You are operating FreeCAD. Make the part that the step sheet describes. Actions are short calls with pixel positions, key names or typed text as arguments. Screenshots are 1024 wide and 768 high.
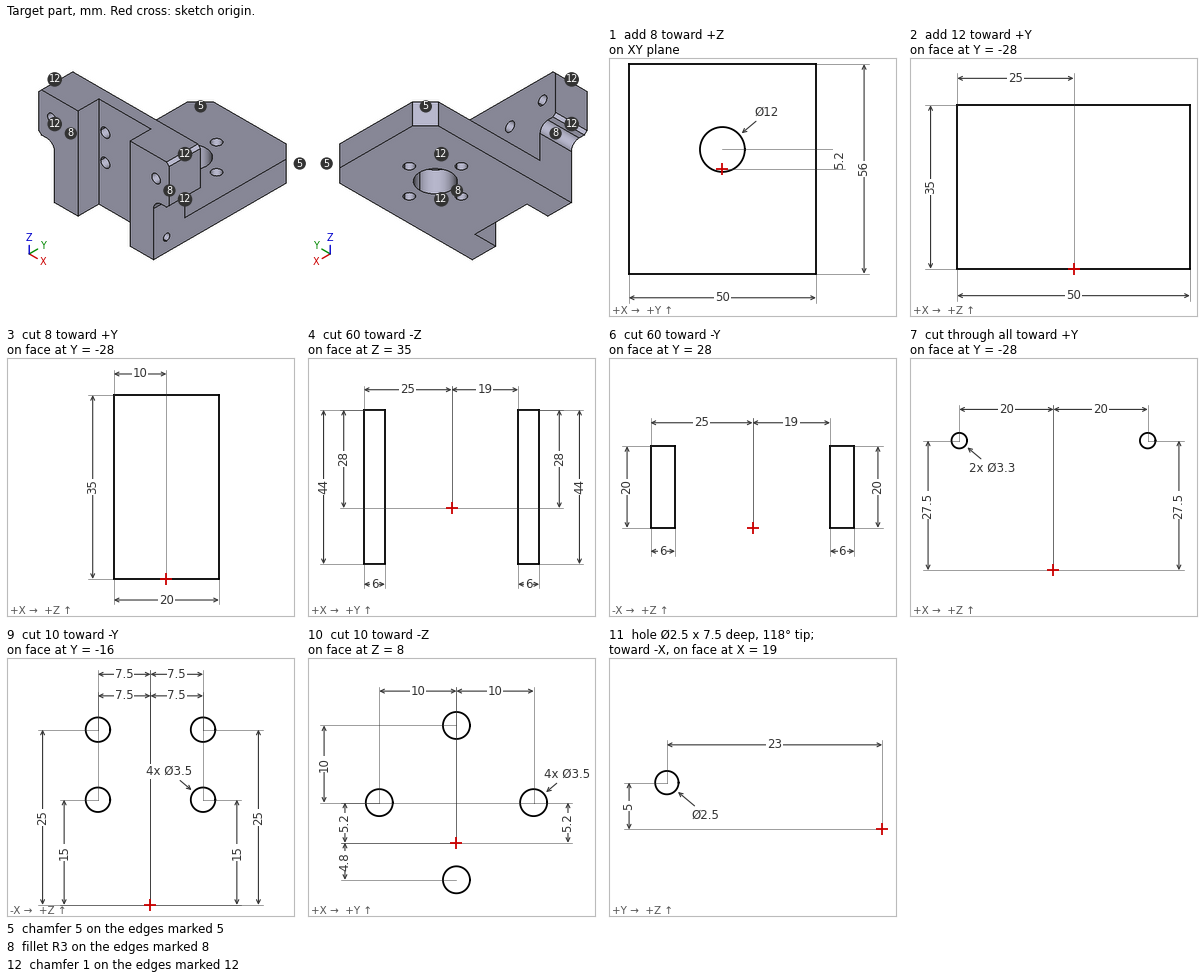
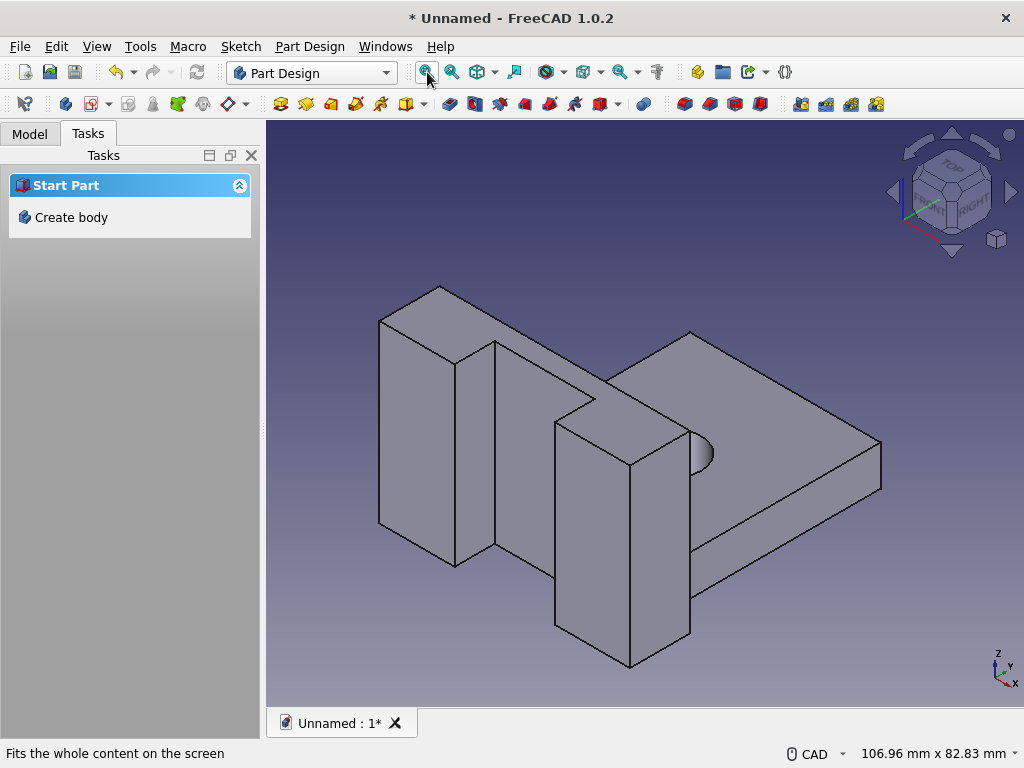
key(2)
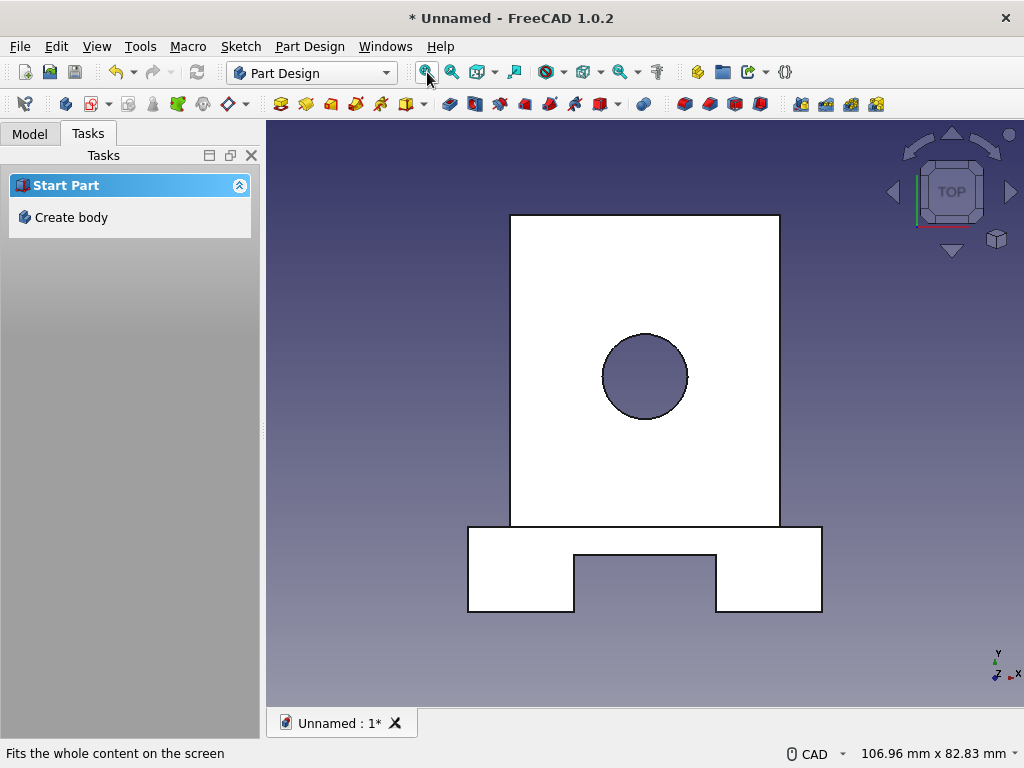
key(1)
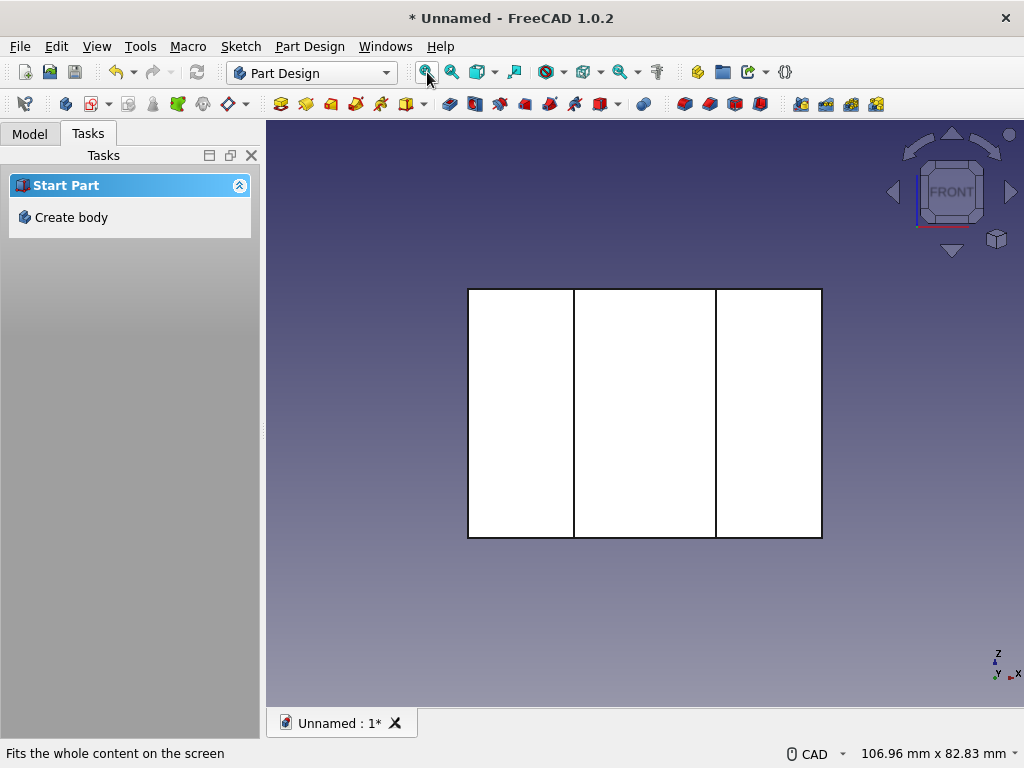
key(3)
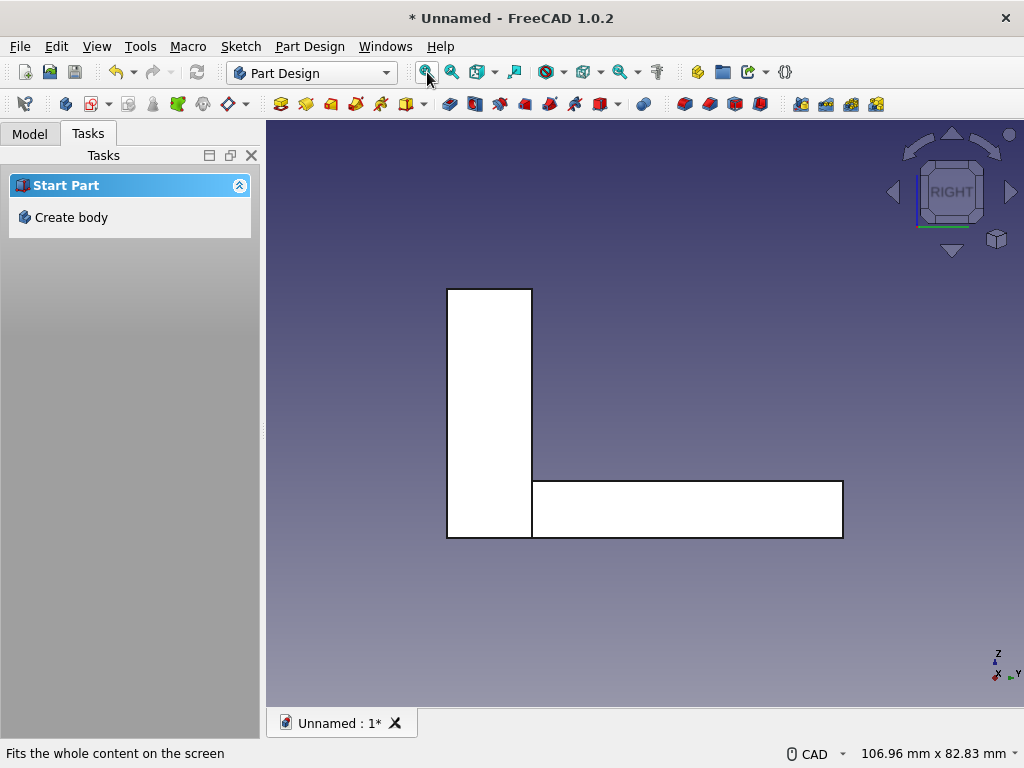
click(843, 508)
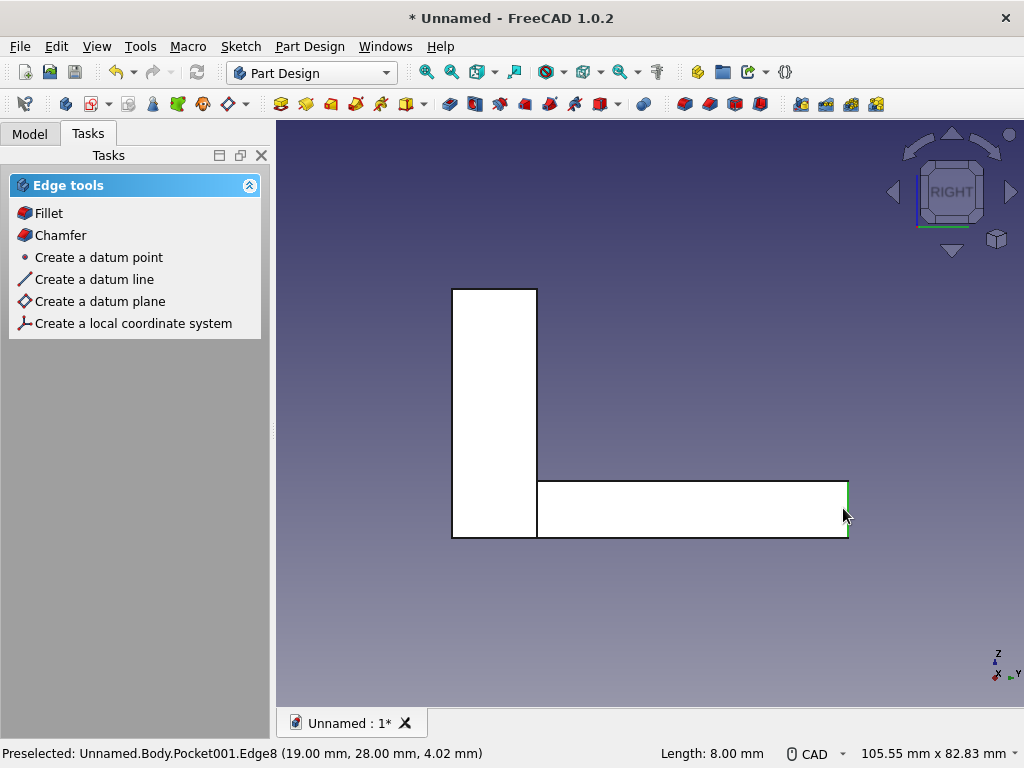
key(5)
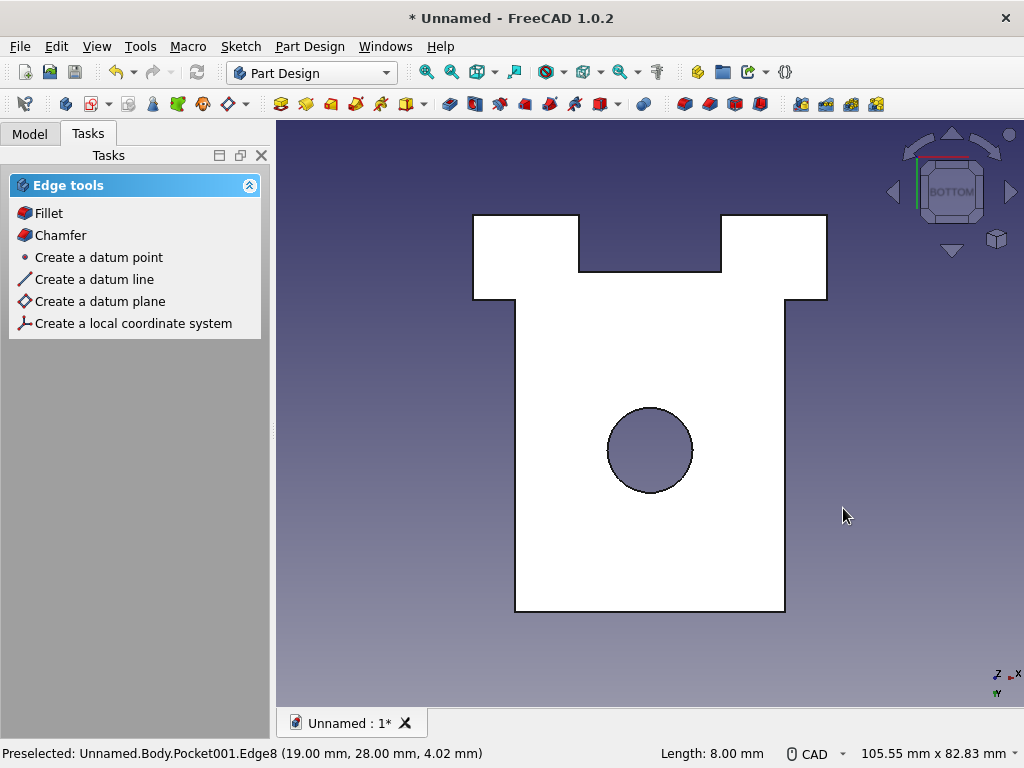
key(4)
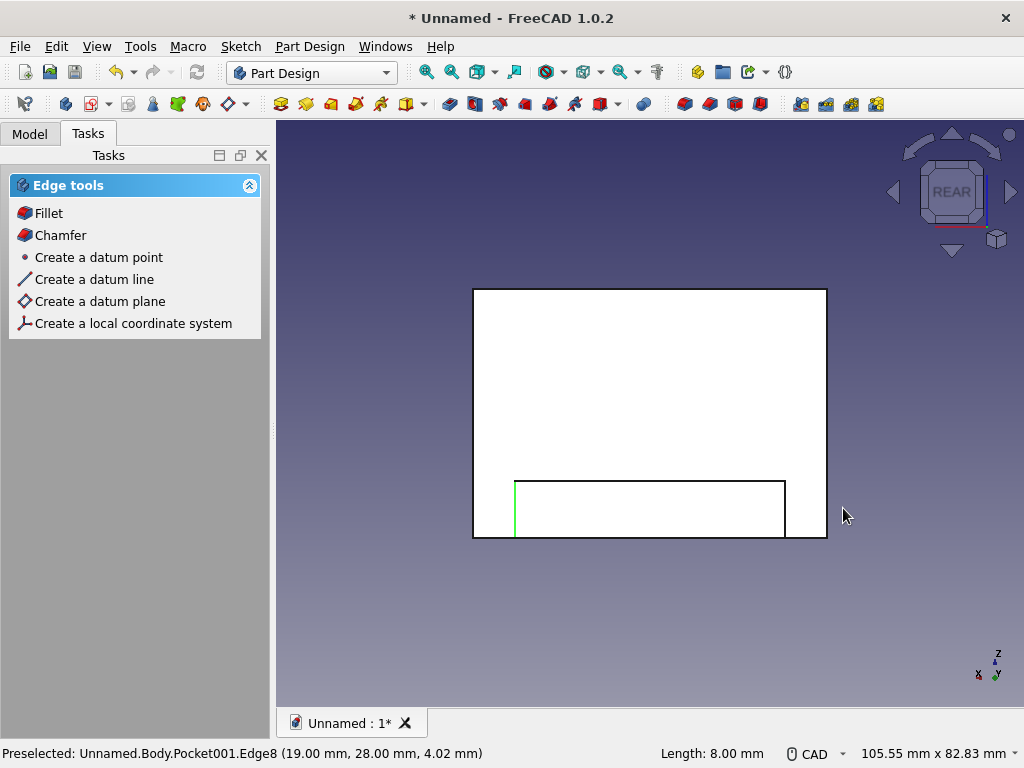
click(785, 508, ctrl)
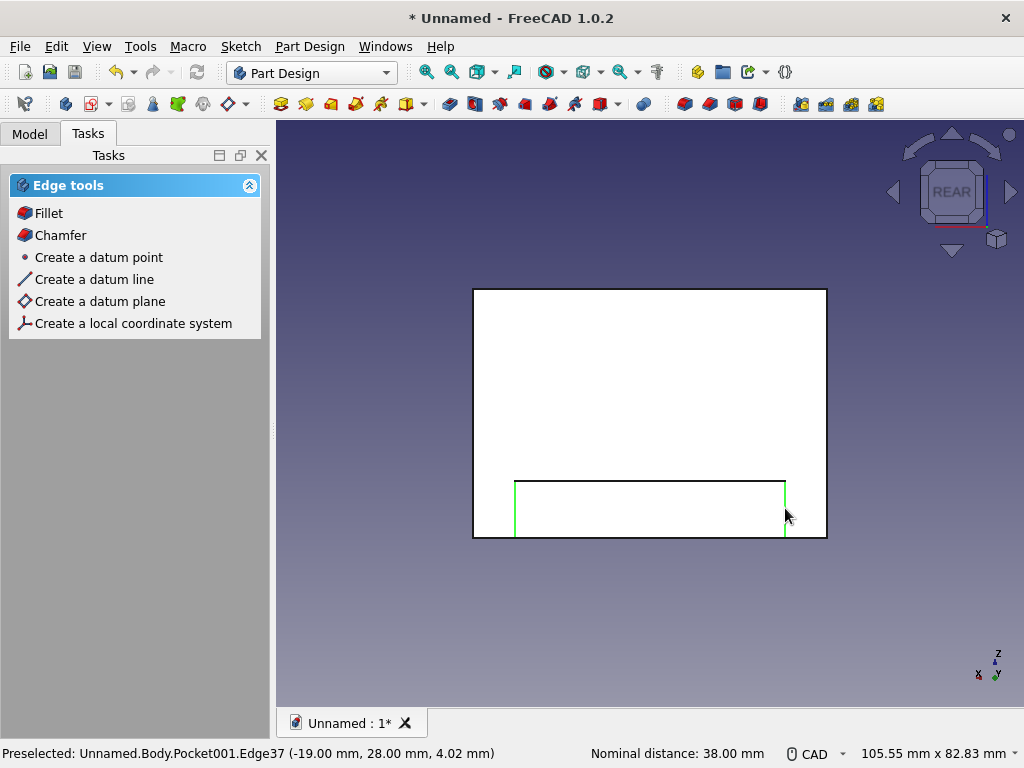
click(710, 104)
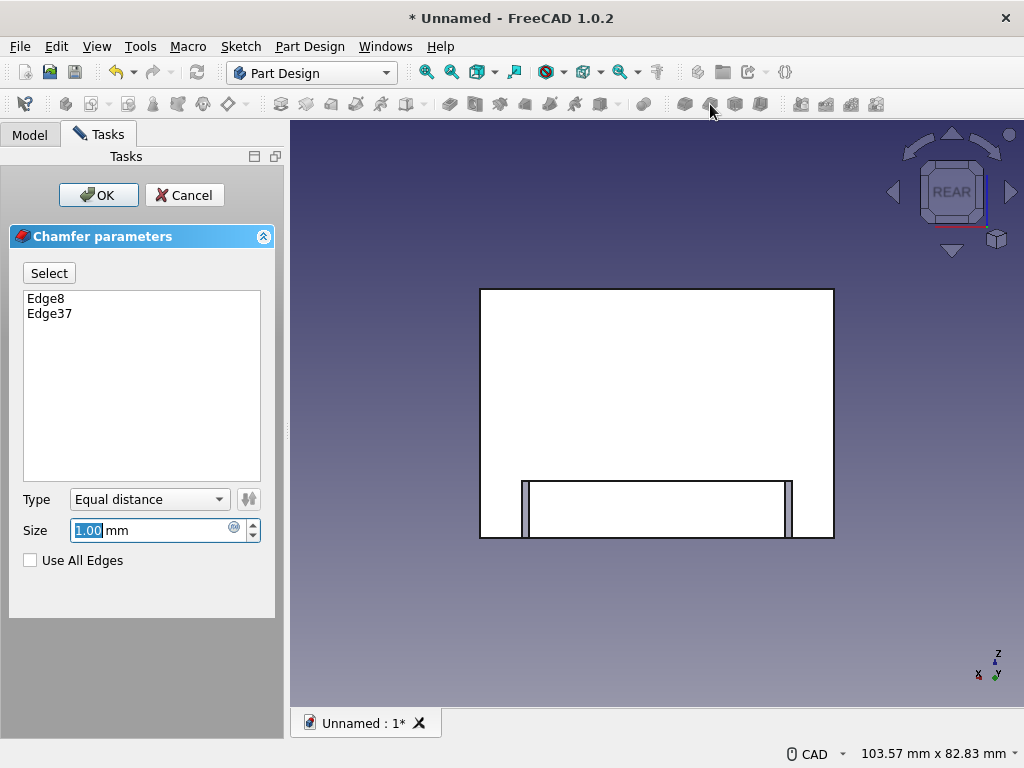
text(5)
key(Tab)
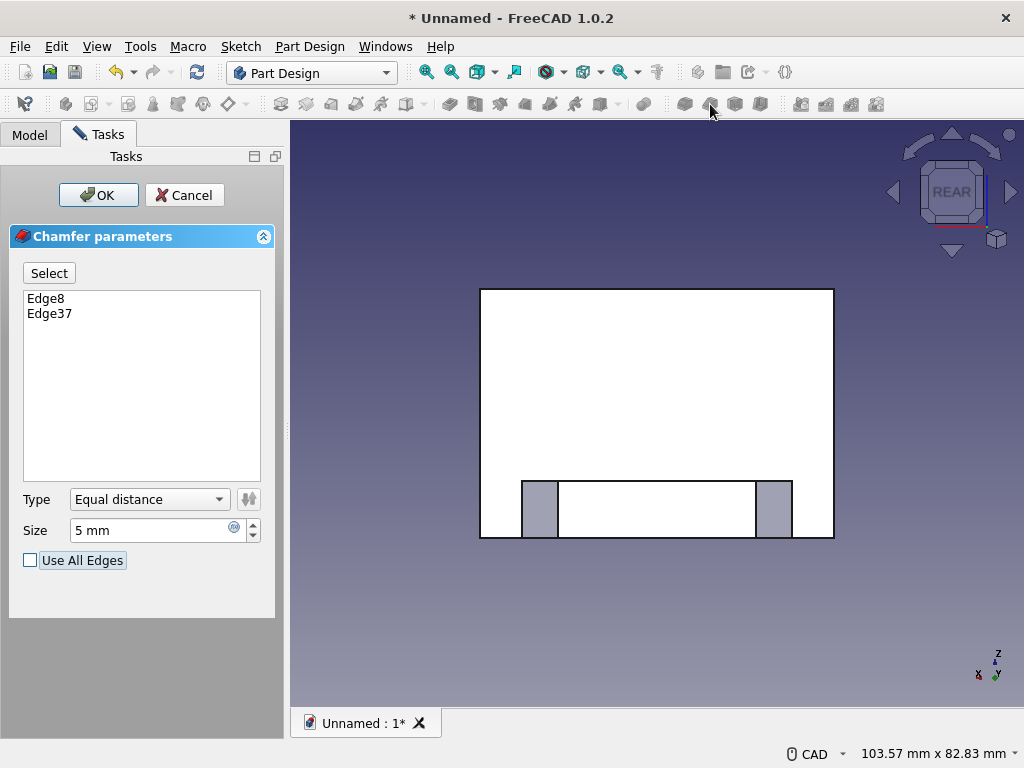
click(99, 195)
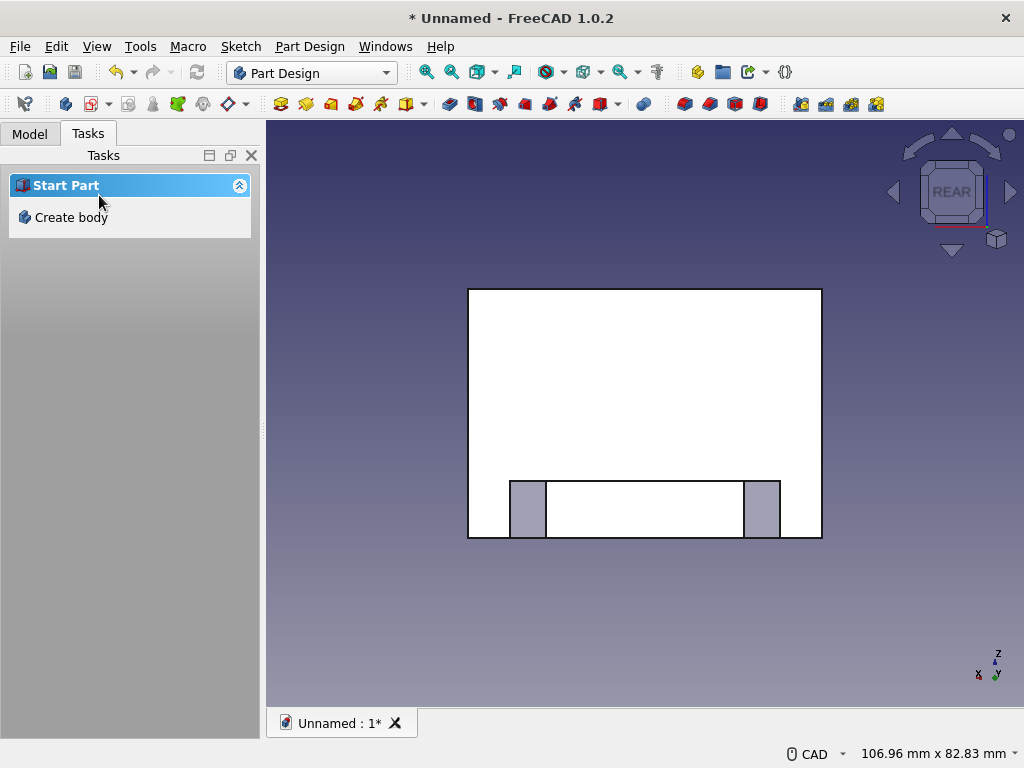
click(588, 508)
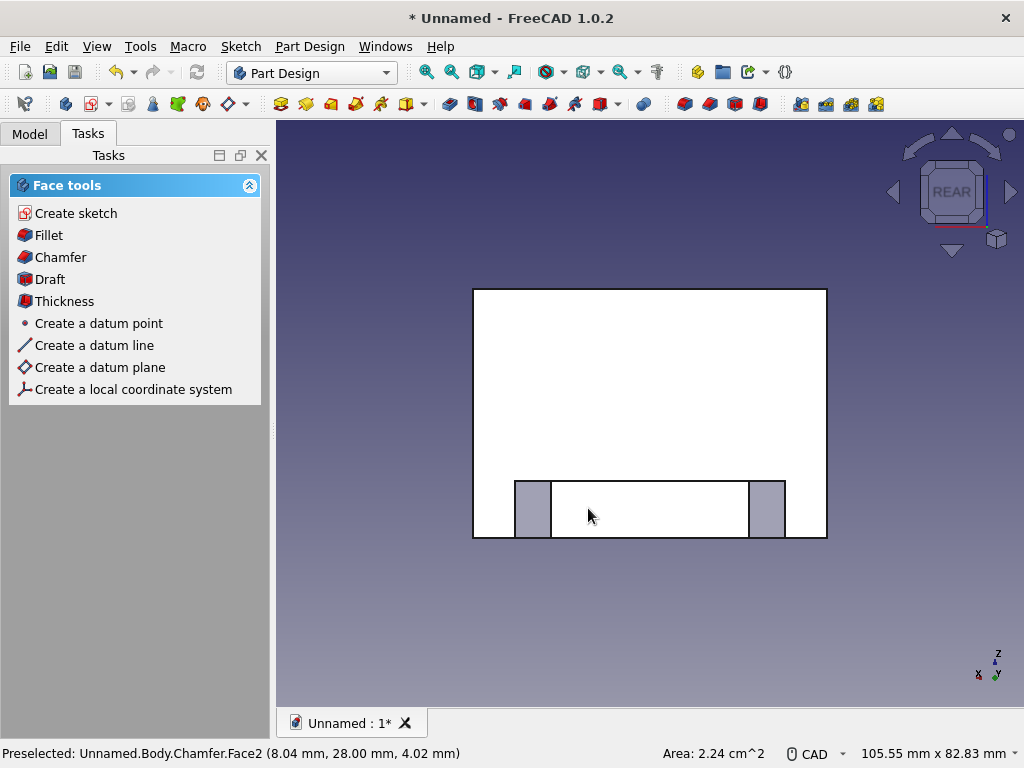
click(90, 104)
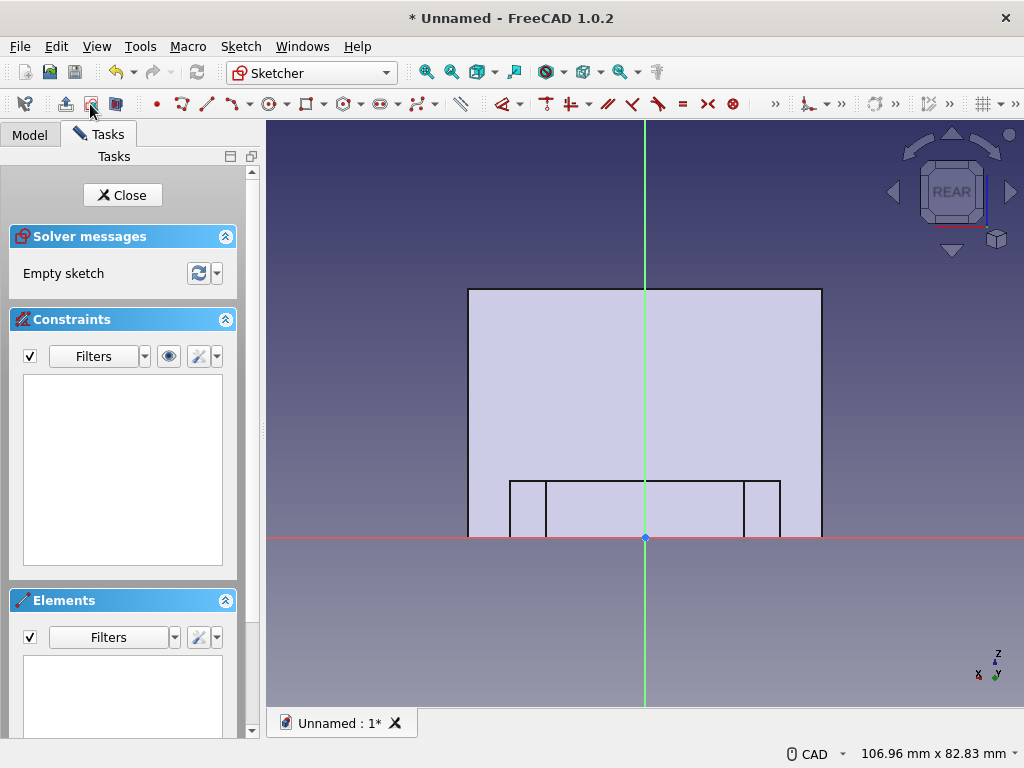
click(306, 104)